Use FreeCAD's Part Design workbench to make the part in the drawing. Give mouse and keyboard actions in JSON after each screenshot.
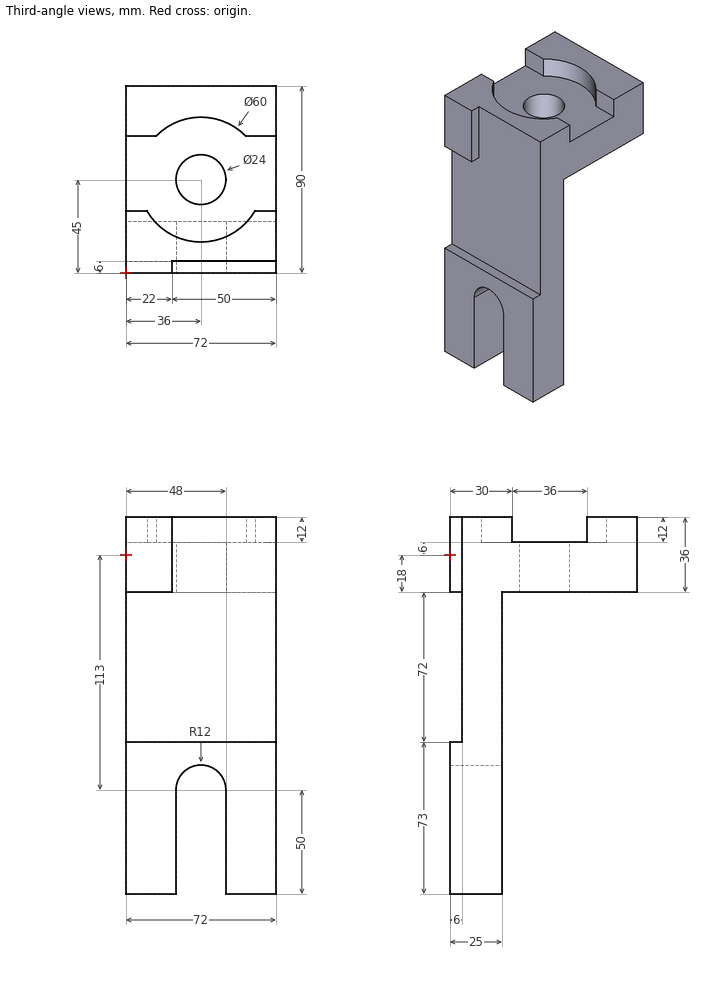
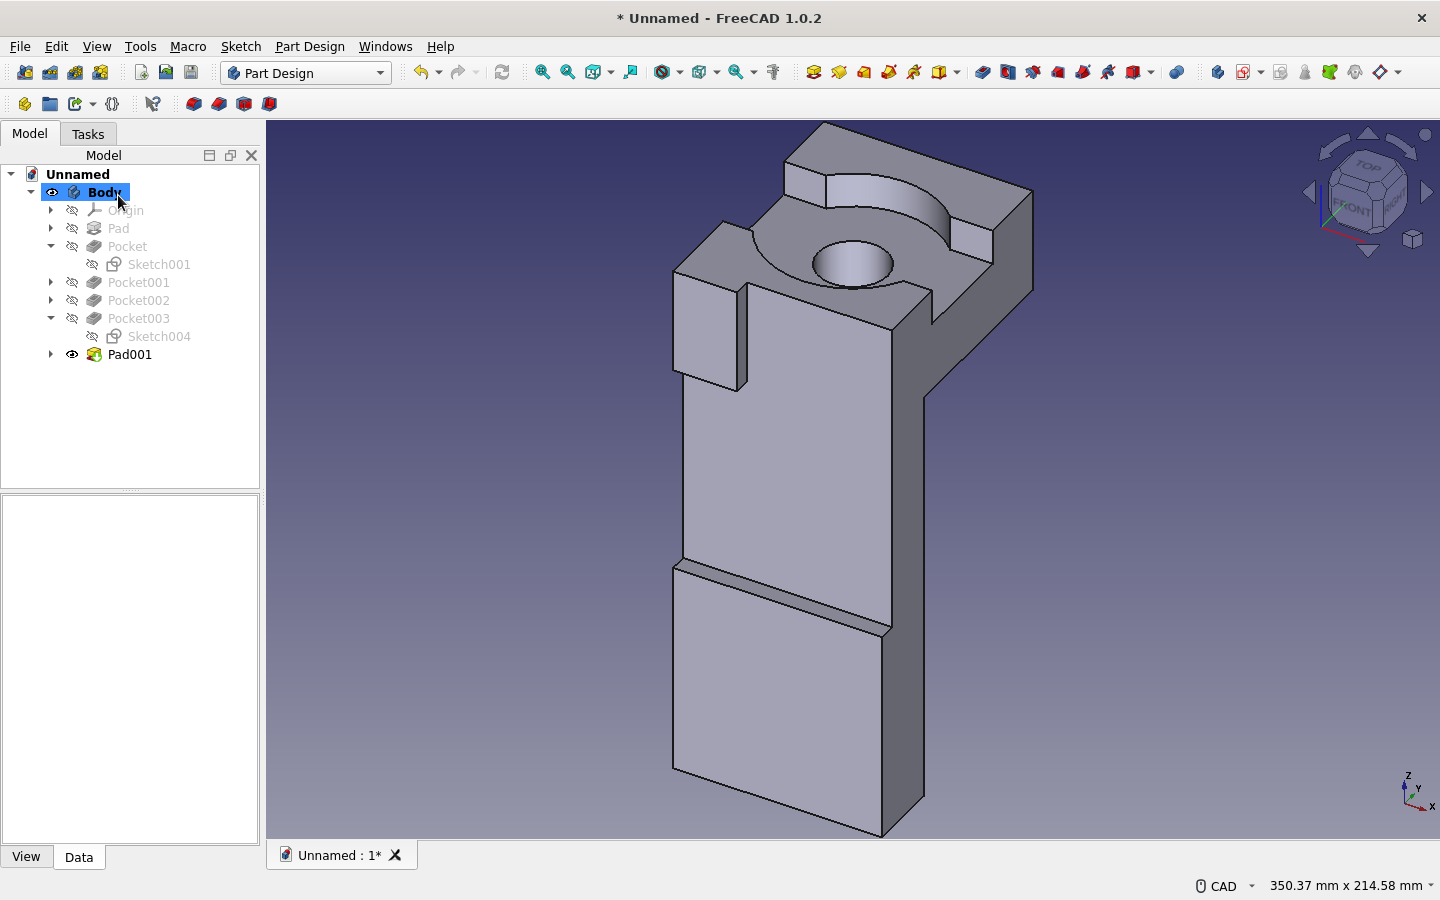
{"action": "key", "text": "4"}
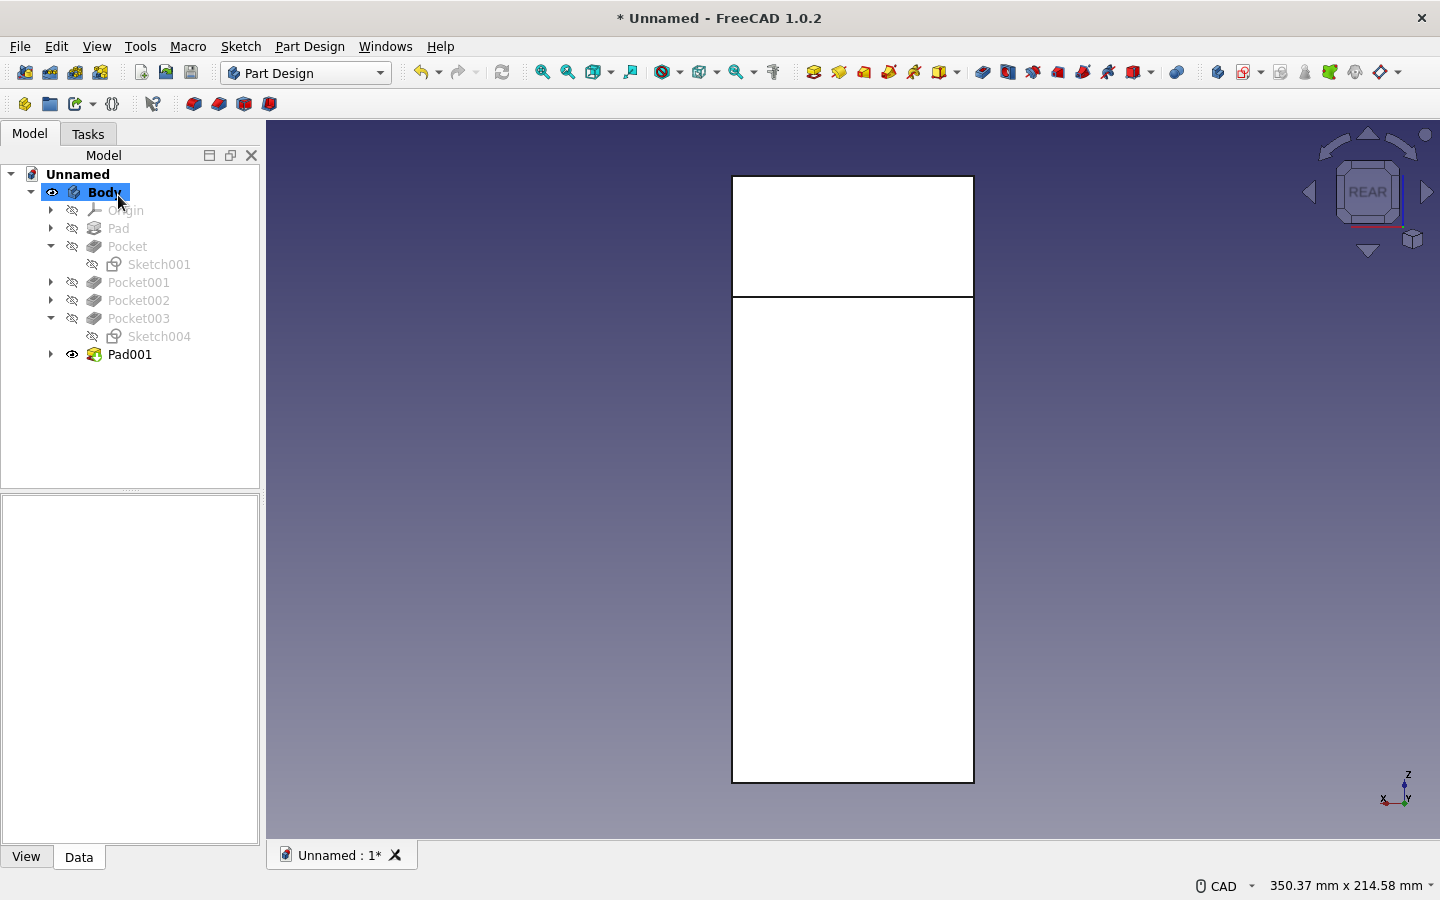
{"action": "left_click", "coordinate": [853, 469]}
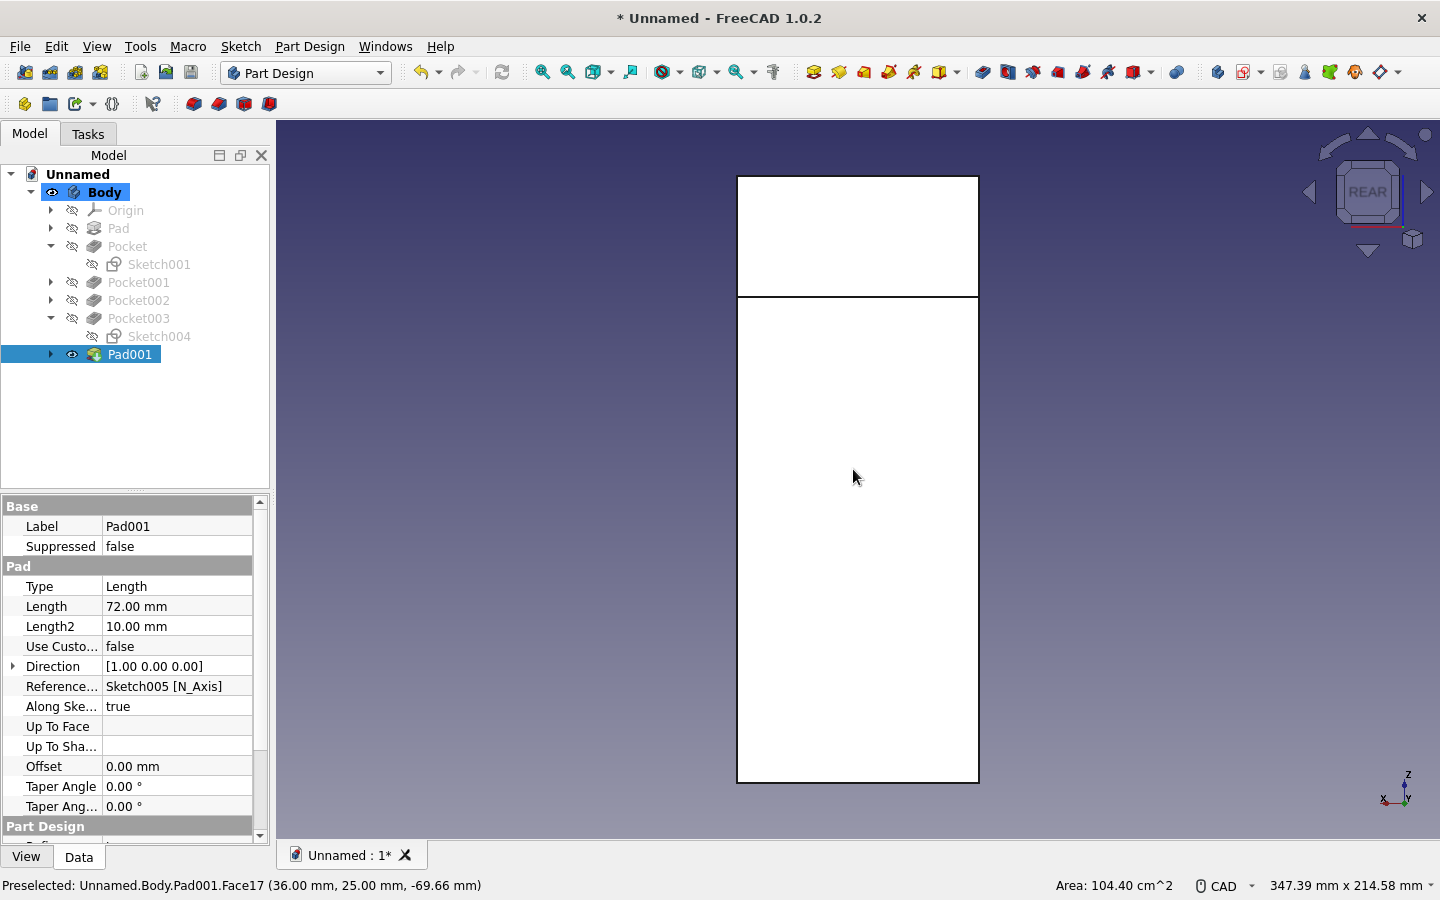
{"action": "left_click", "coordinate": [1242, 72]}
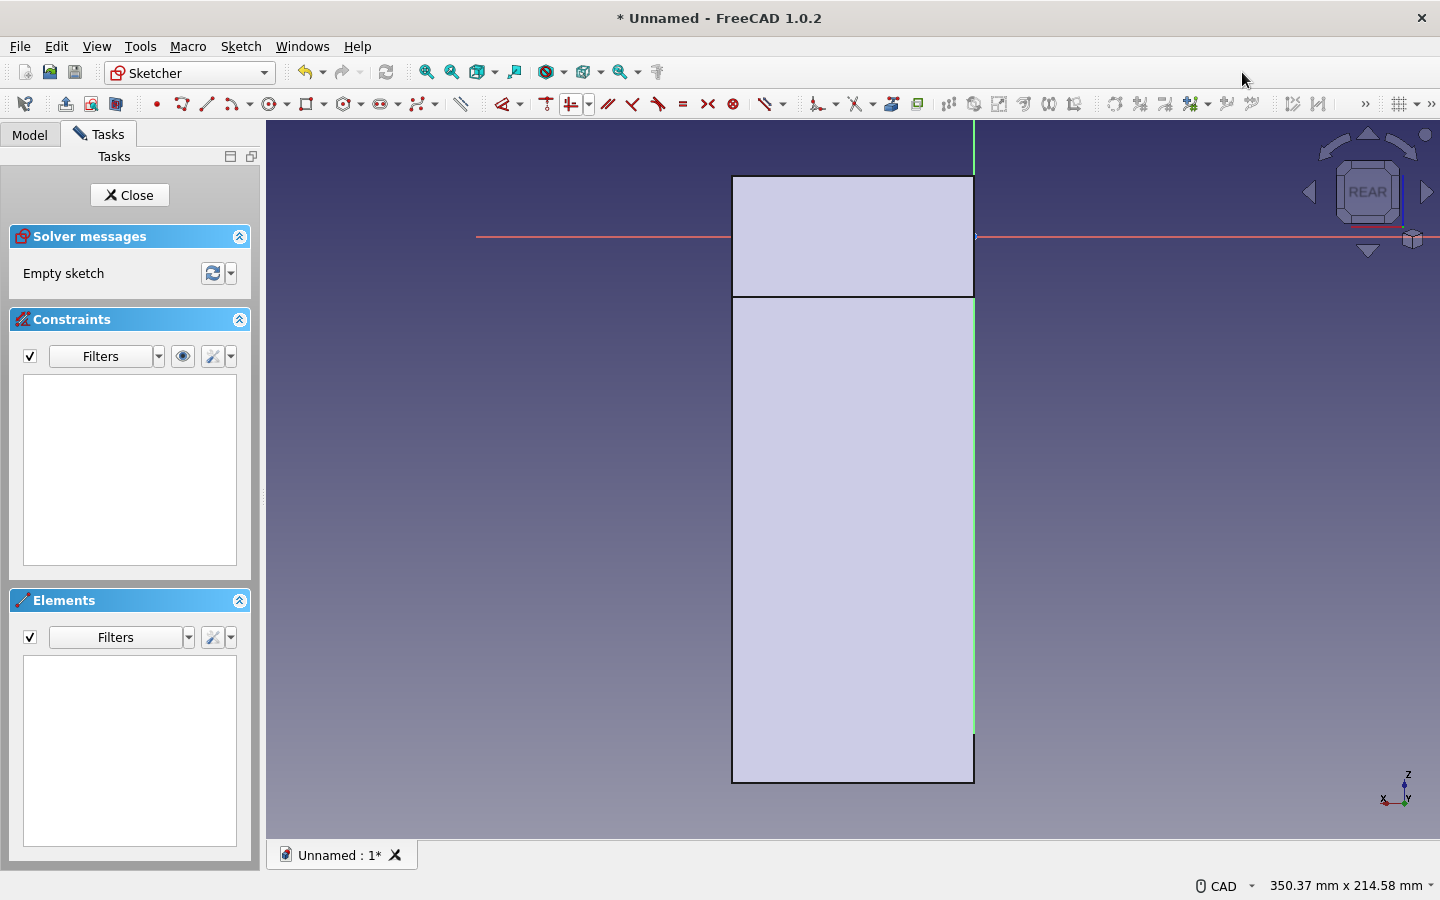
{"action": "scroll", "coordinate": [909, 811], "scroll_direction": "up", "scroll_amount": 4}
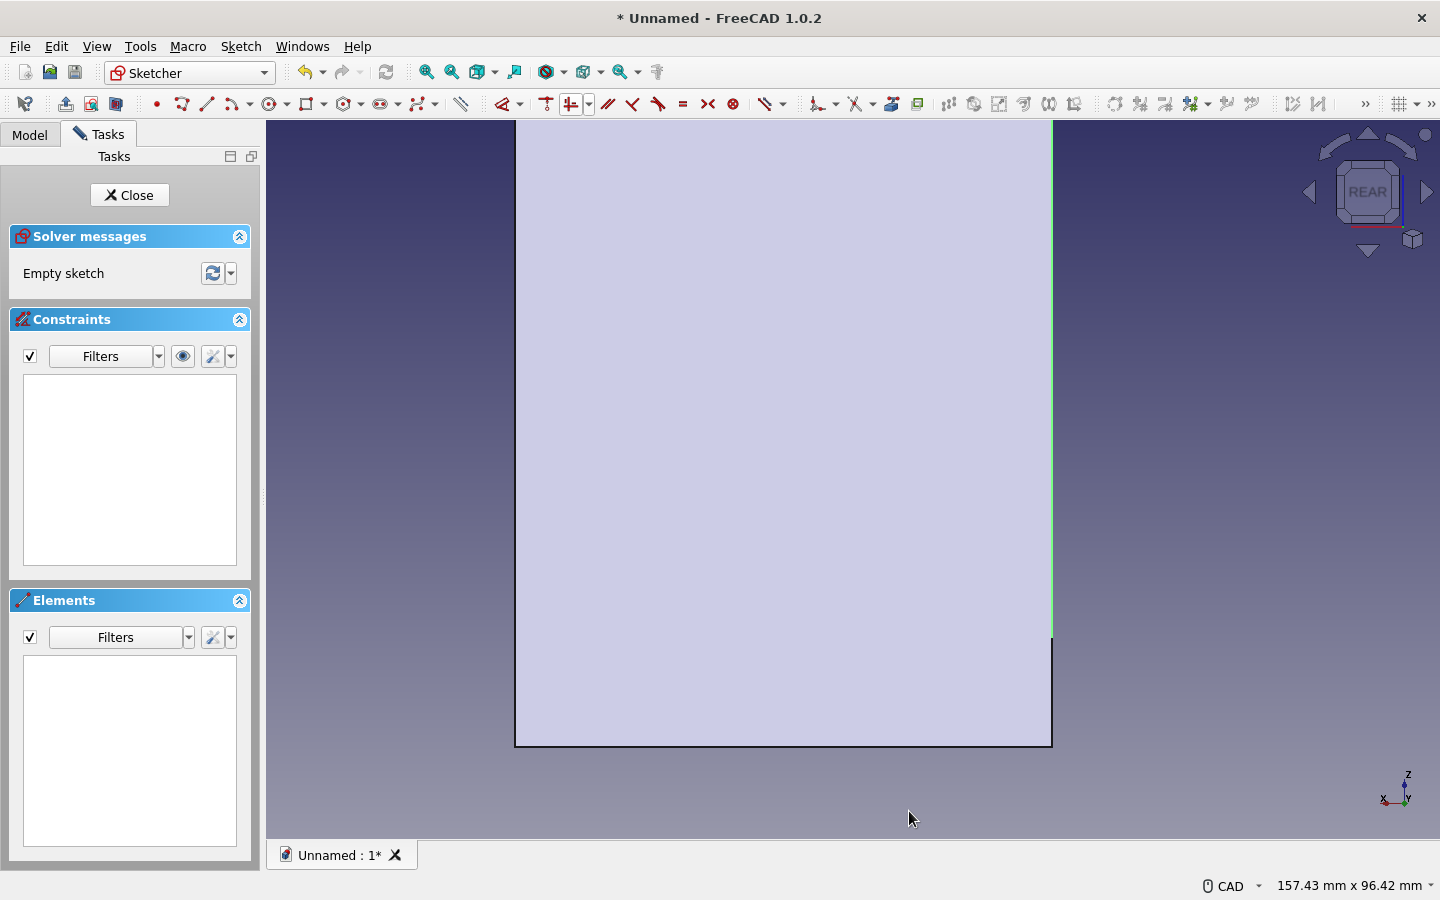
{"action": "key", "text": "g m"}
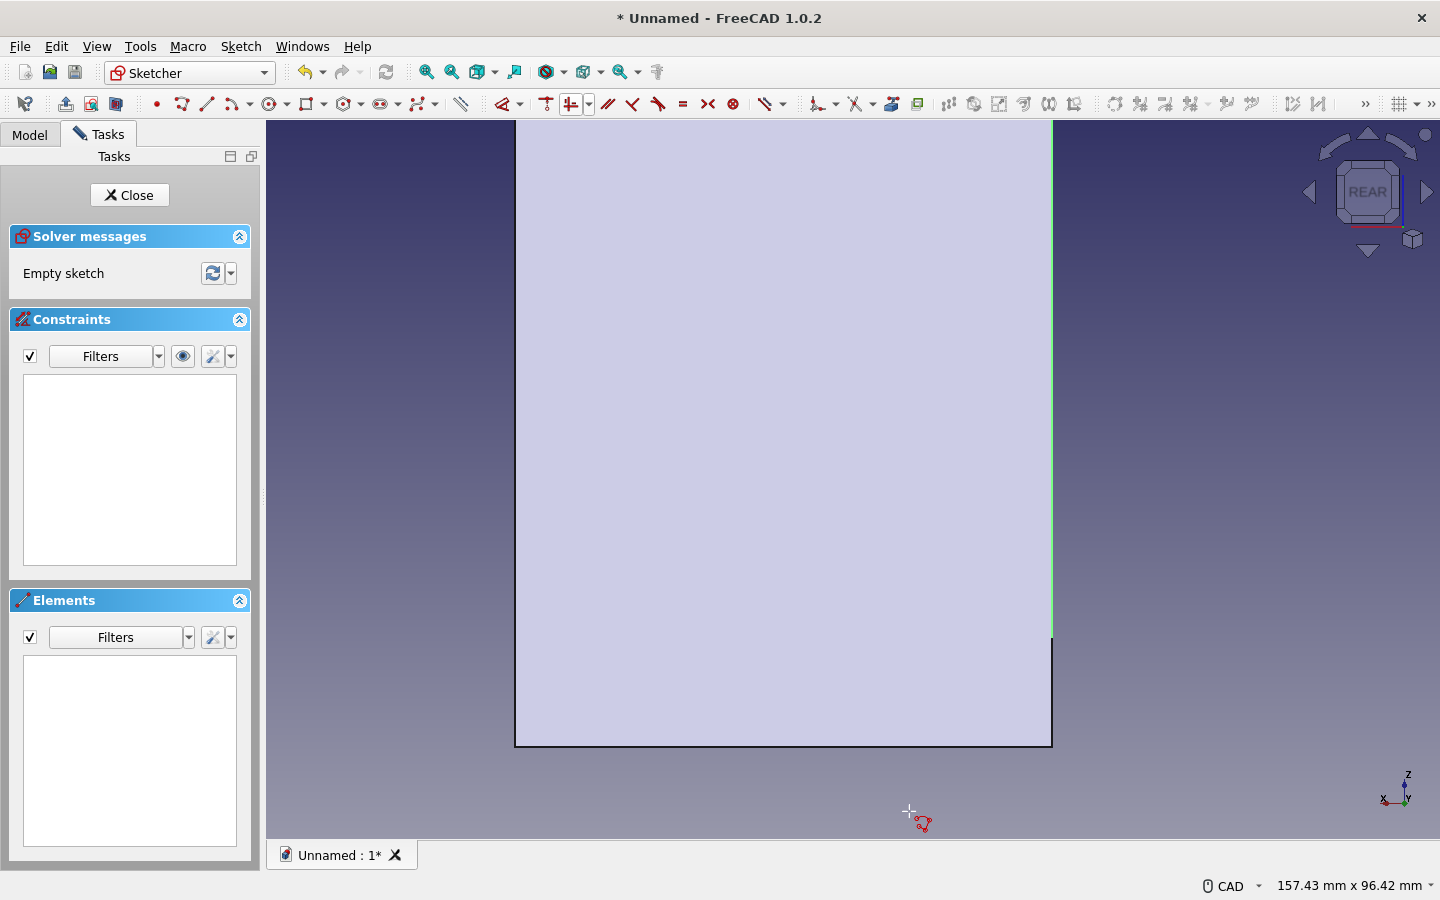
{"action": "left_click", "coordinate": [694, 374]}
{"action": "left_click", "coordinate": [694, 747]}
{"action": "left_click", "coordinate": [873, 747]}
{"action": "left_click", "coordinate": [873, 374]}
{"action": "right_click", "coordinate": [873, 374]}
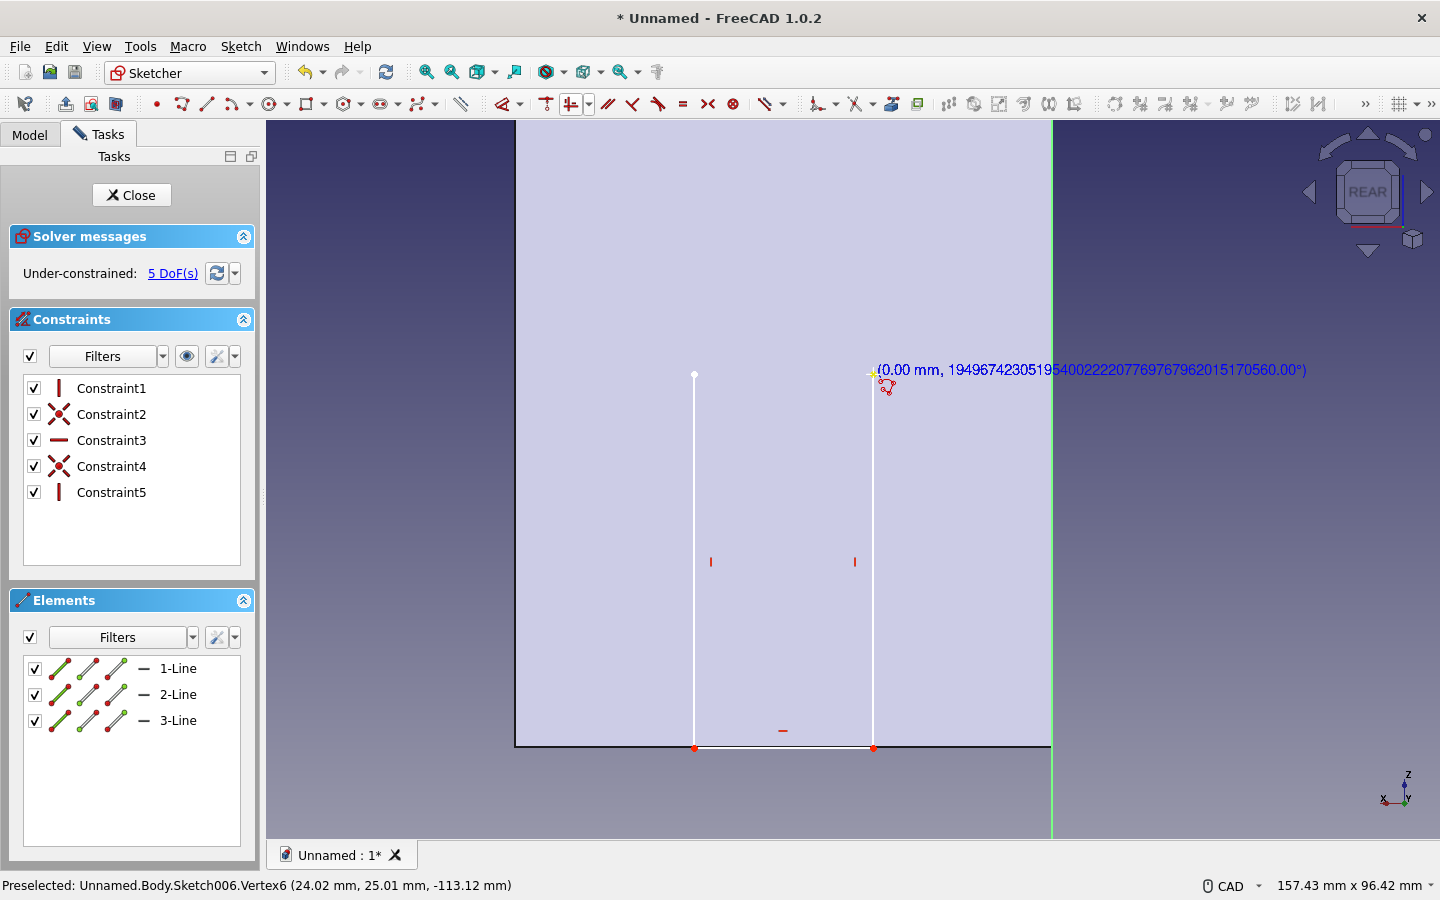
{"action": "key", "text": "g 3 a"}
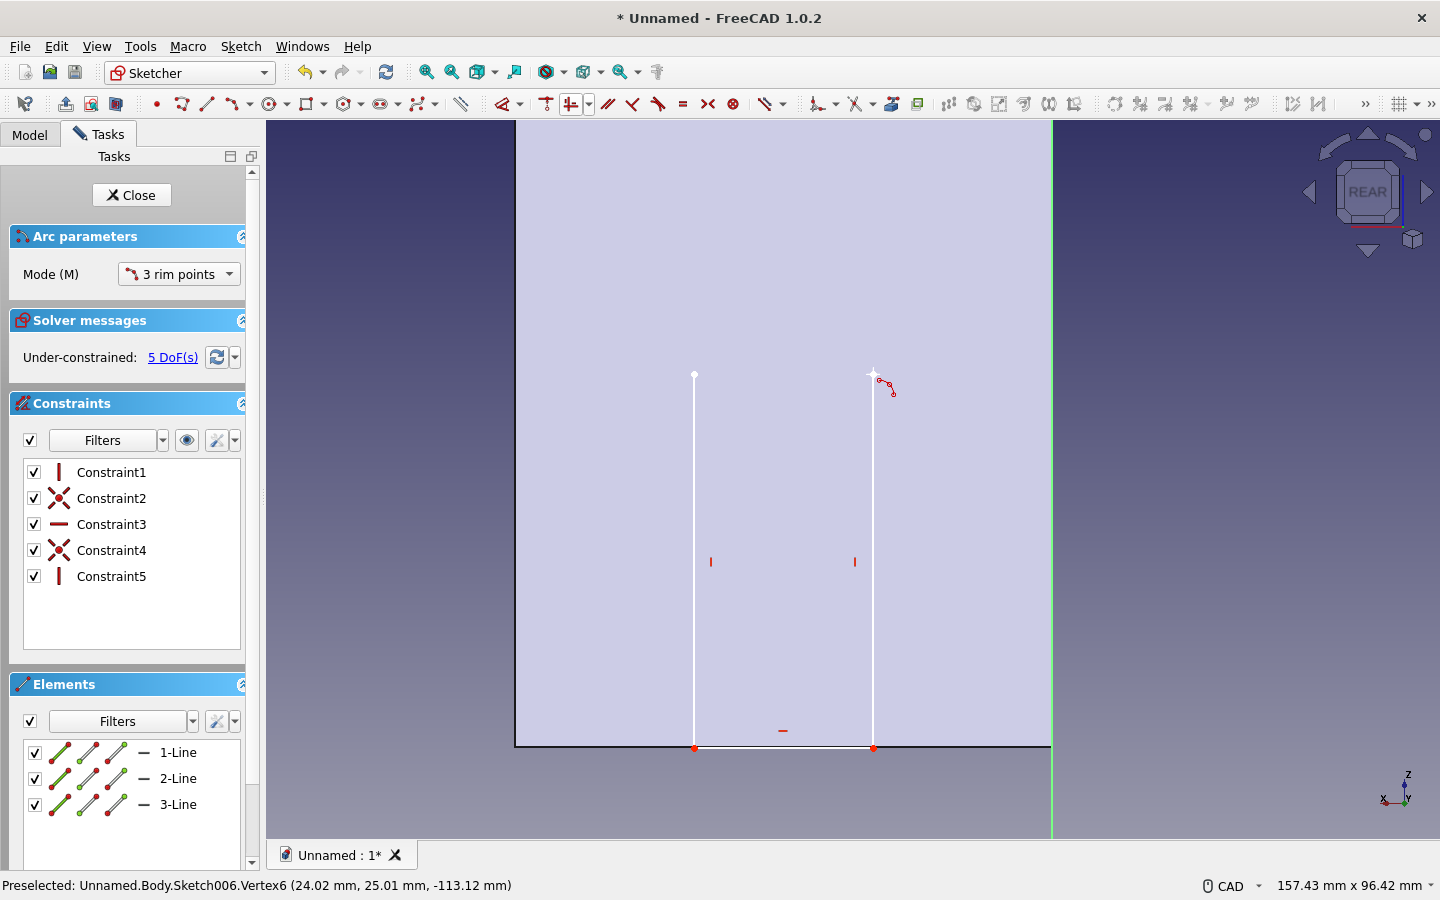
{"action": "left_click", "coordinate": [873, 375]}
{"action": "left_click", "coordinate": [694, 375]}
{"action": "left_click", "coordinate": [784, 285]}
{"action": "key", "text": "Escape"}